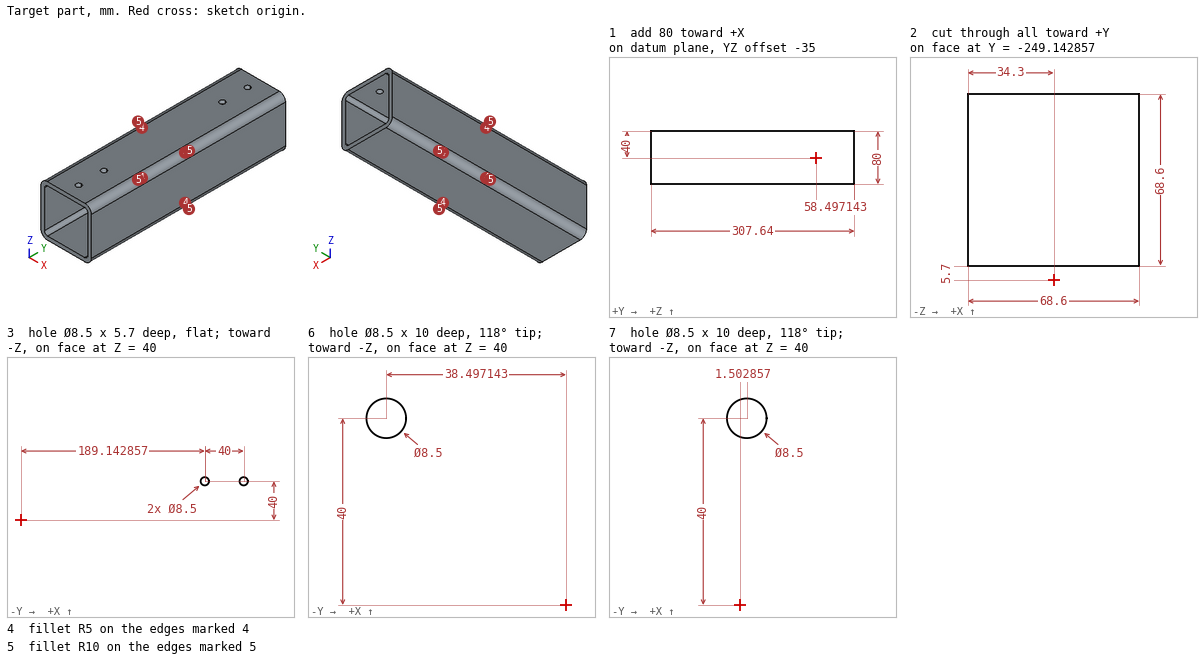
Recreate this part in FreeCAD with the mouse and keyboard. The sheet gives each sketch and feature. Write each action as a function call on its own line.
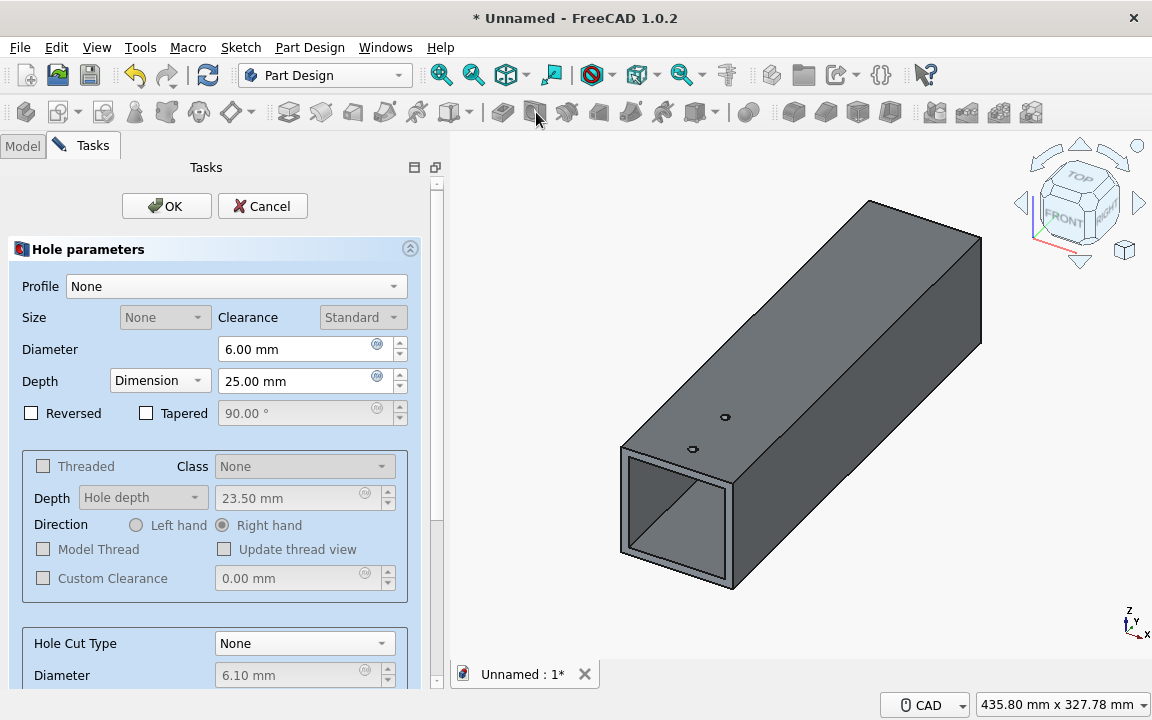
triple_click(305, 349)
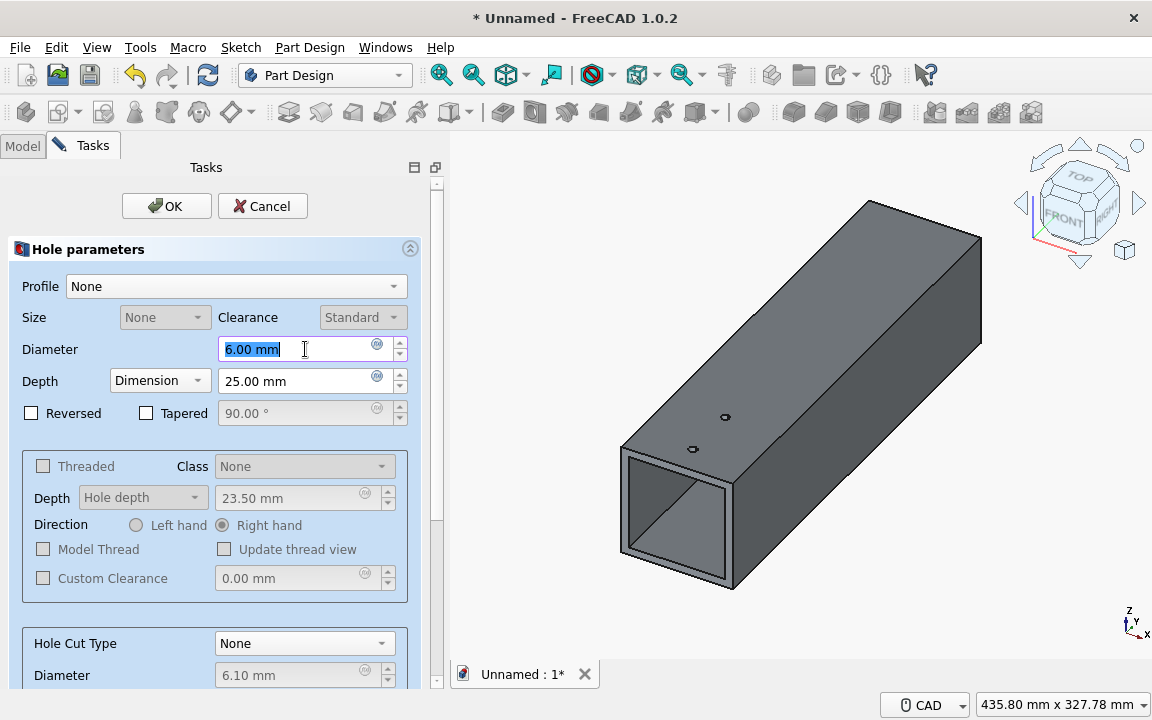
text(8.5)
key(Tab)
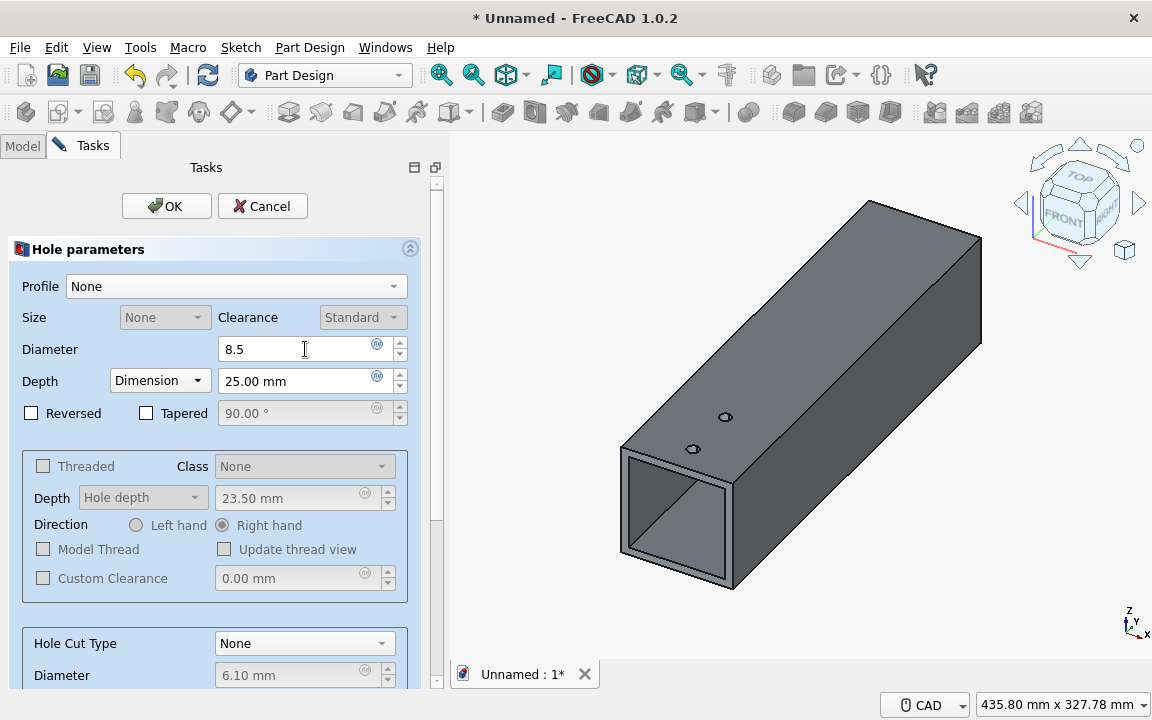
triple_click(305, 381)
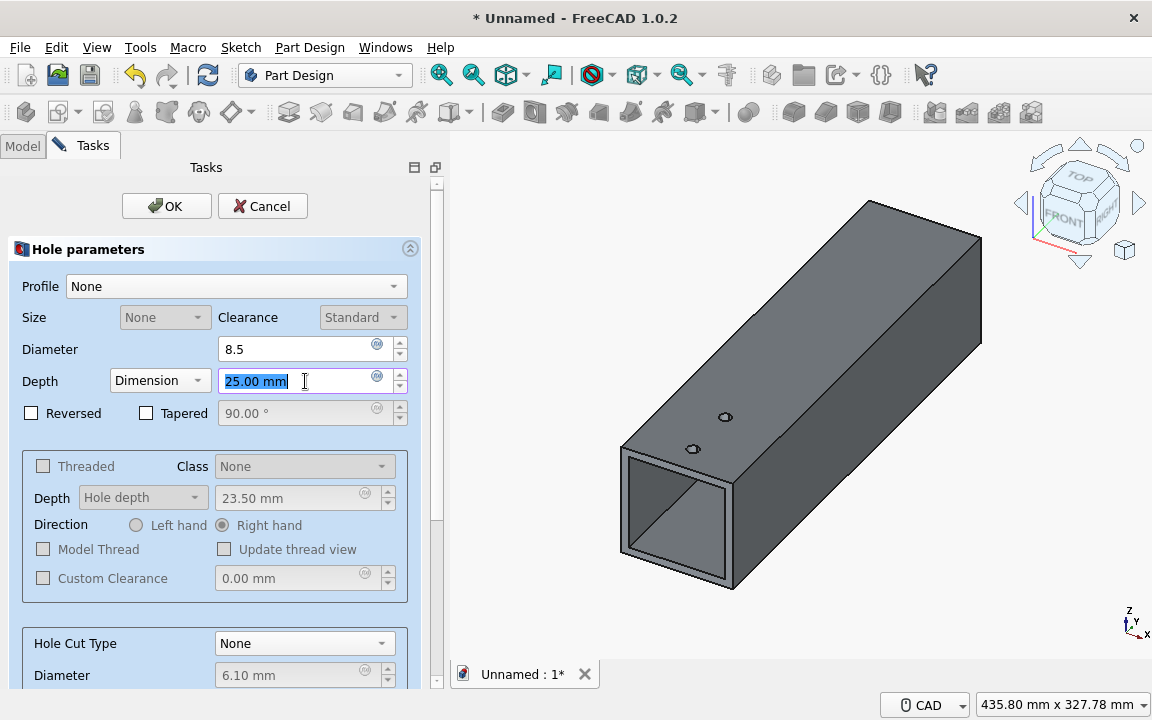
text(5.7)
key(Tab)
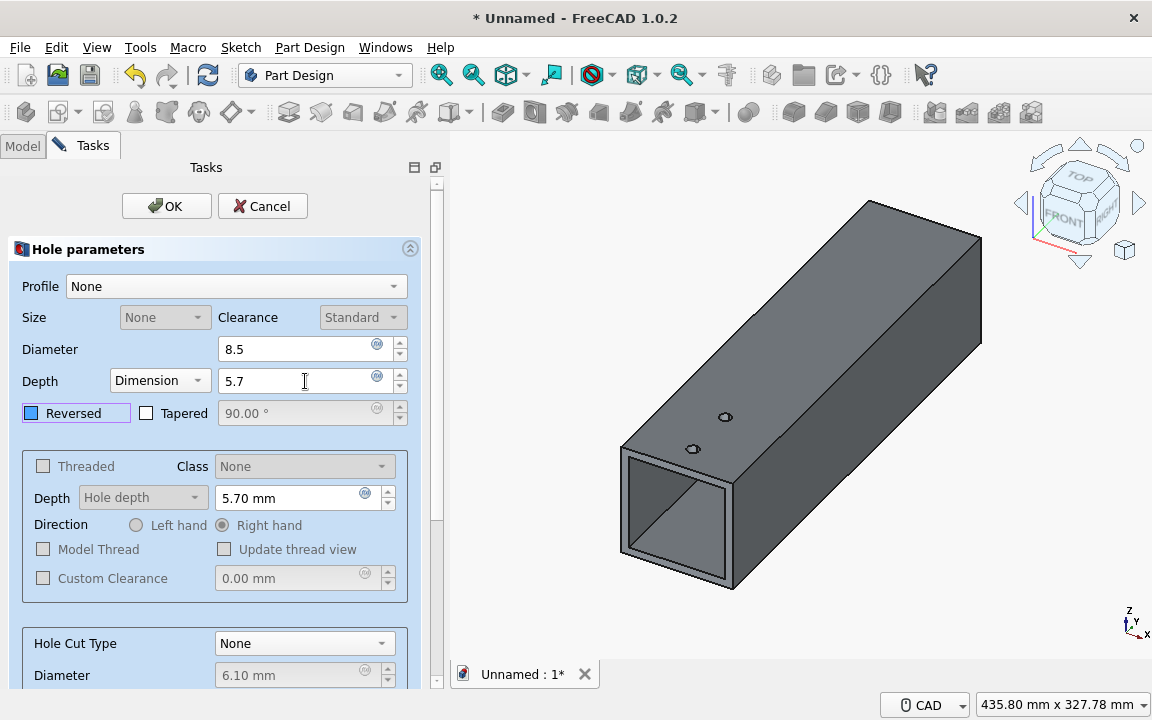
scroll(437, 432, down, 4)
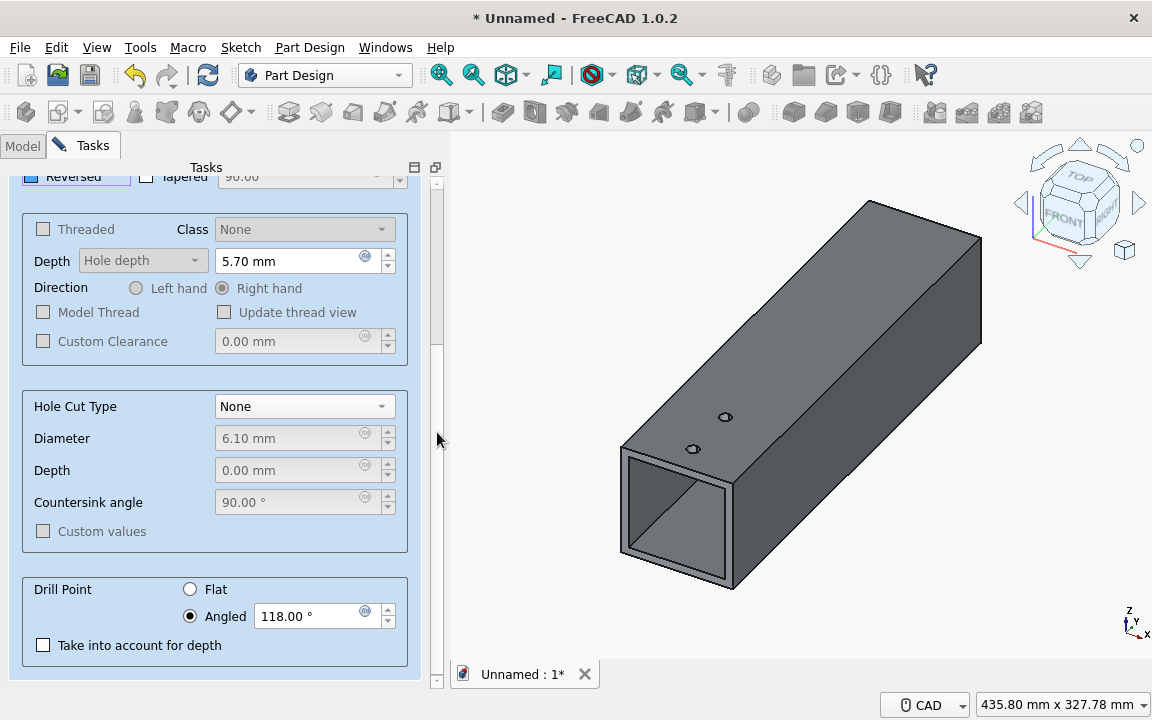
click(191, 589)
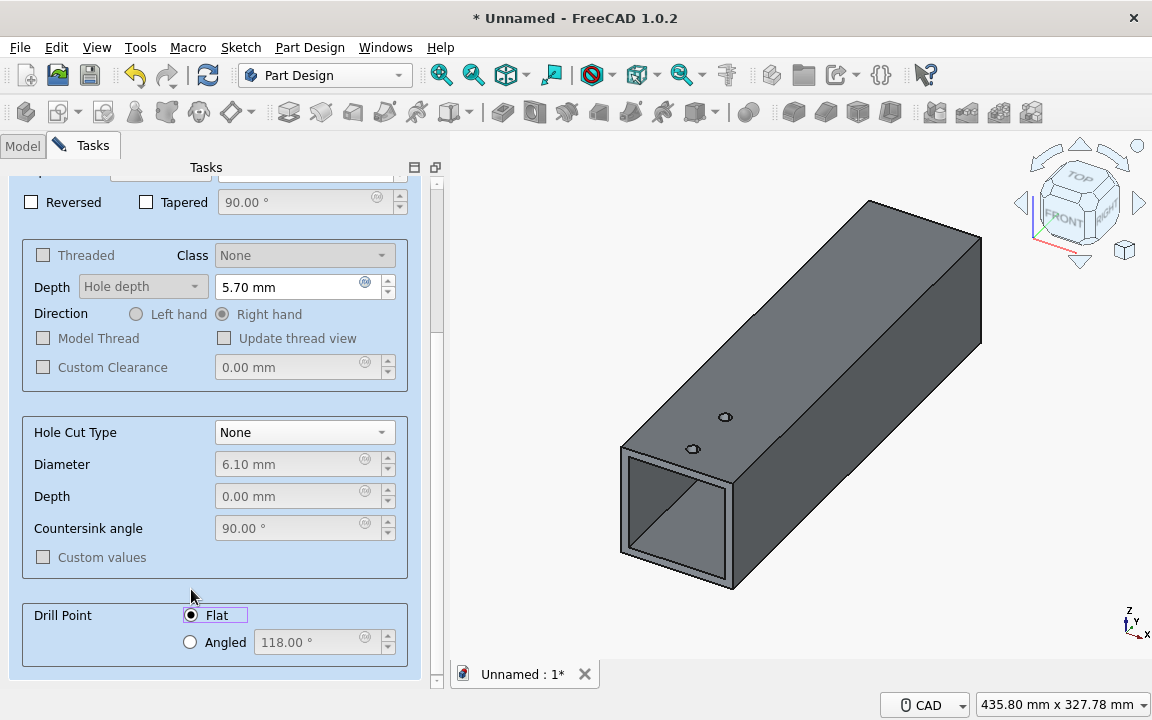
scroll(437, 432, up, 5)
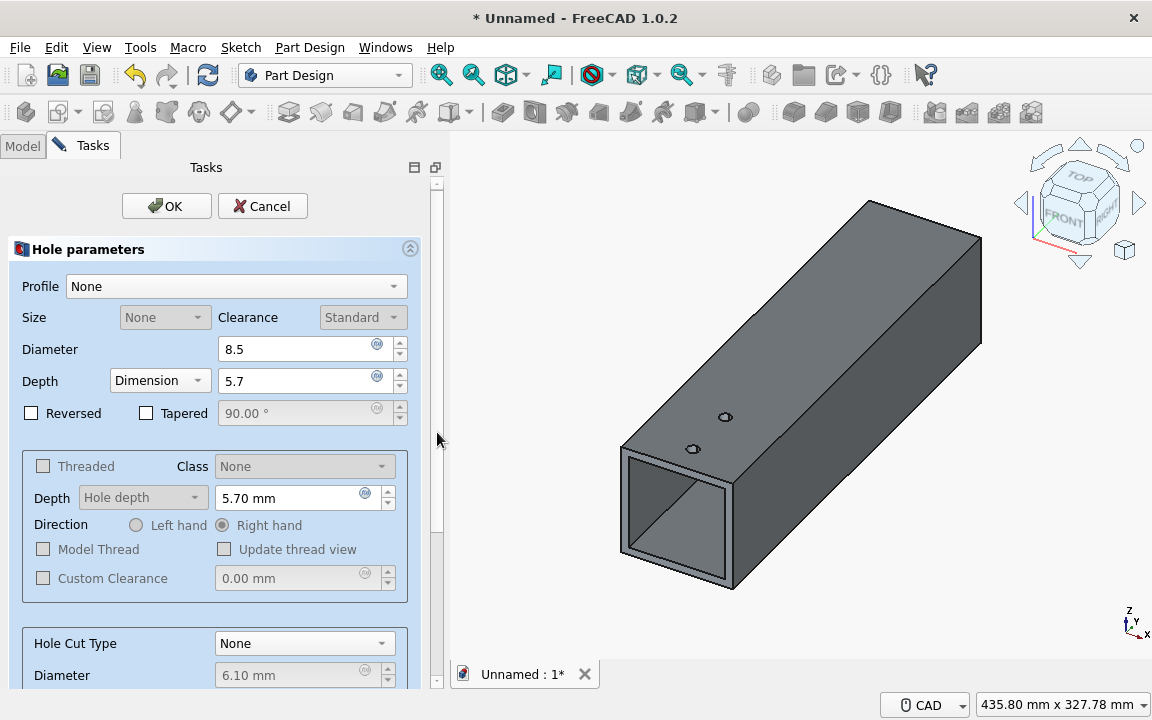
click(167, 206)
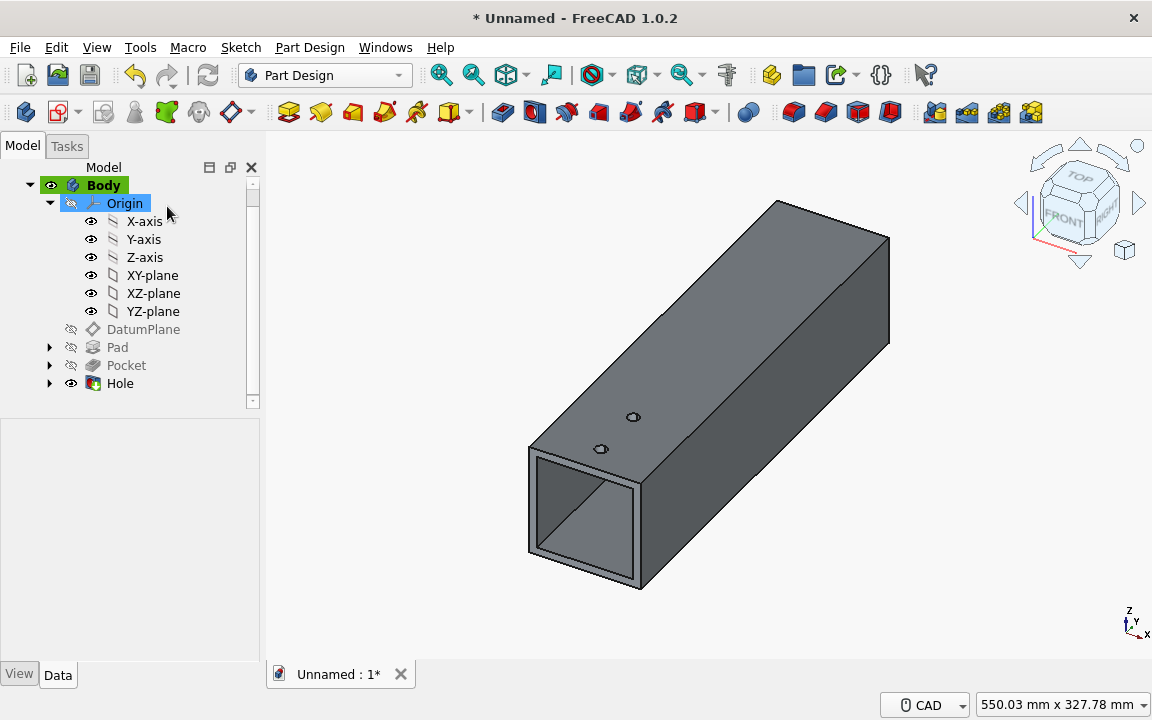
key(0)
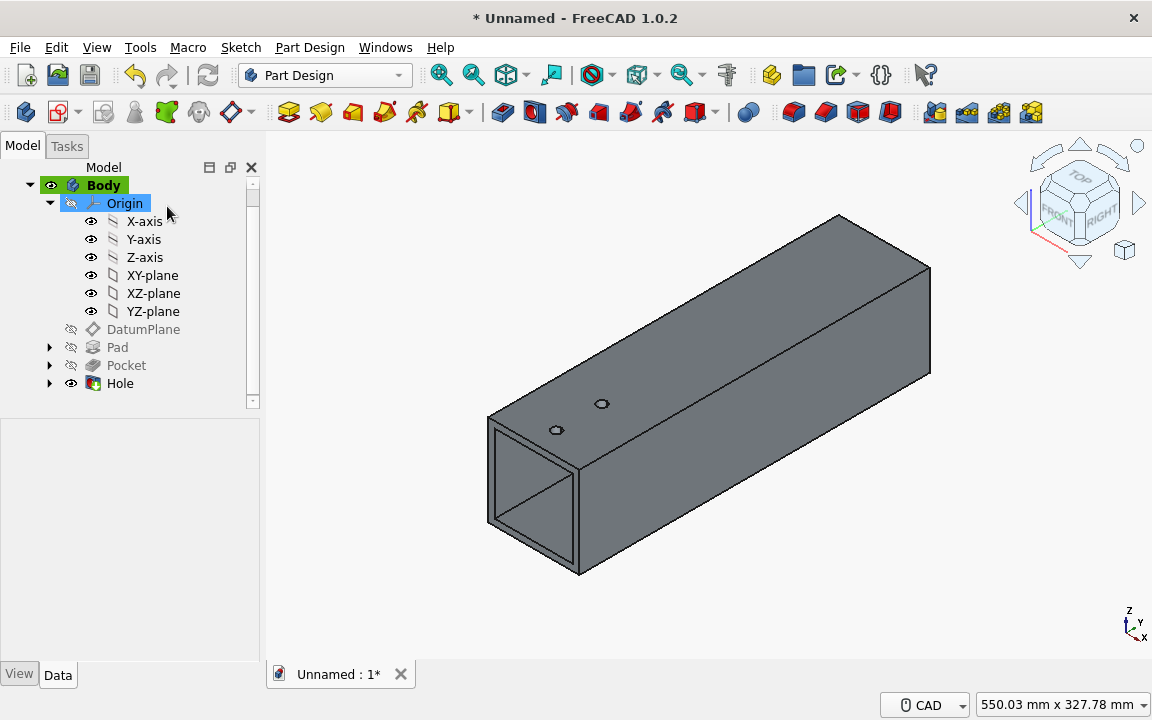
key(2)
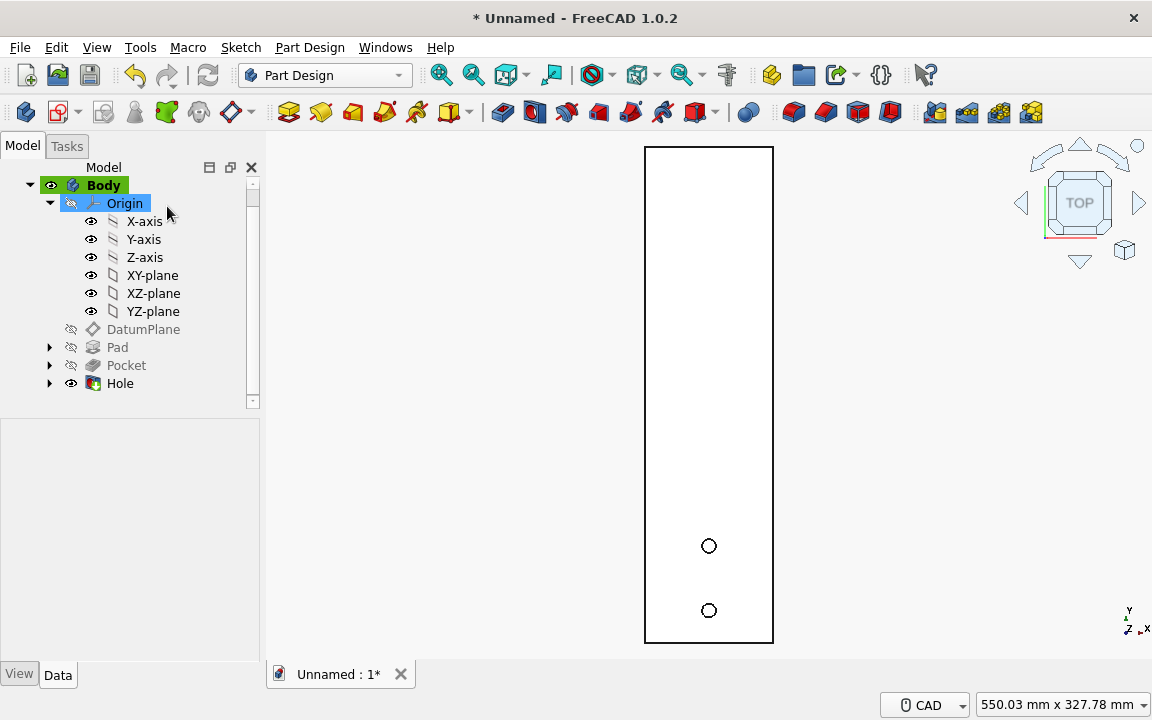
key(1)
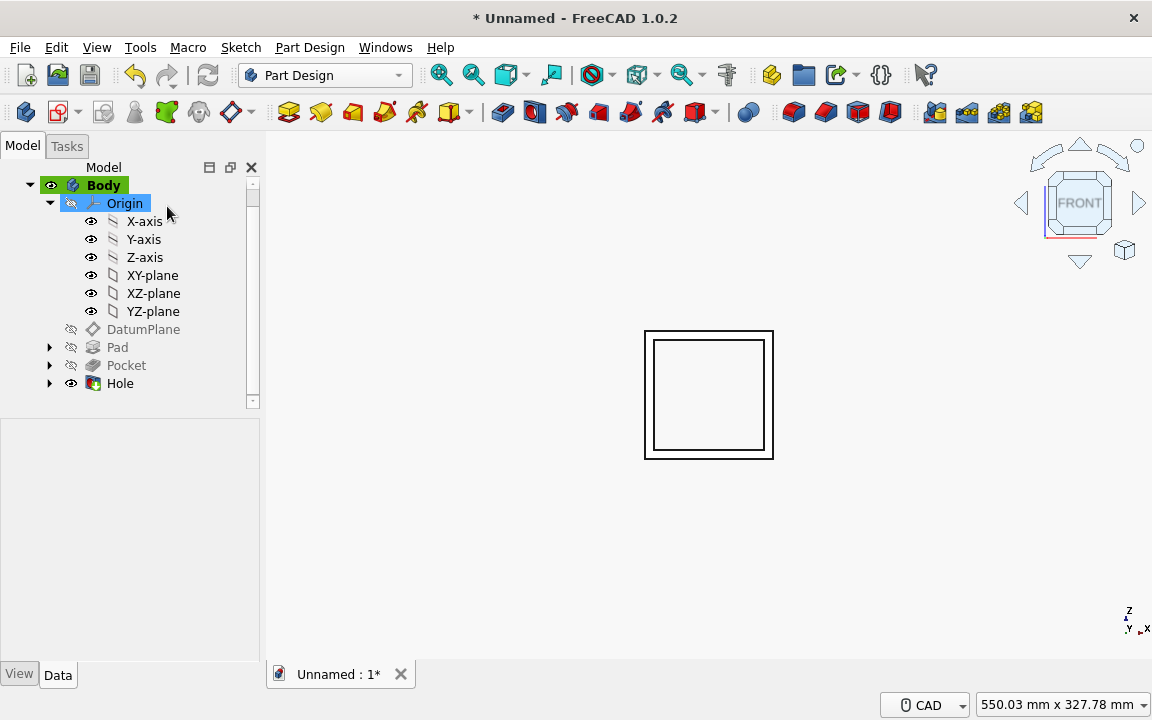
key(v)
key(f)